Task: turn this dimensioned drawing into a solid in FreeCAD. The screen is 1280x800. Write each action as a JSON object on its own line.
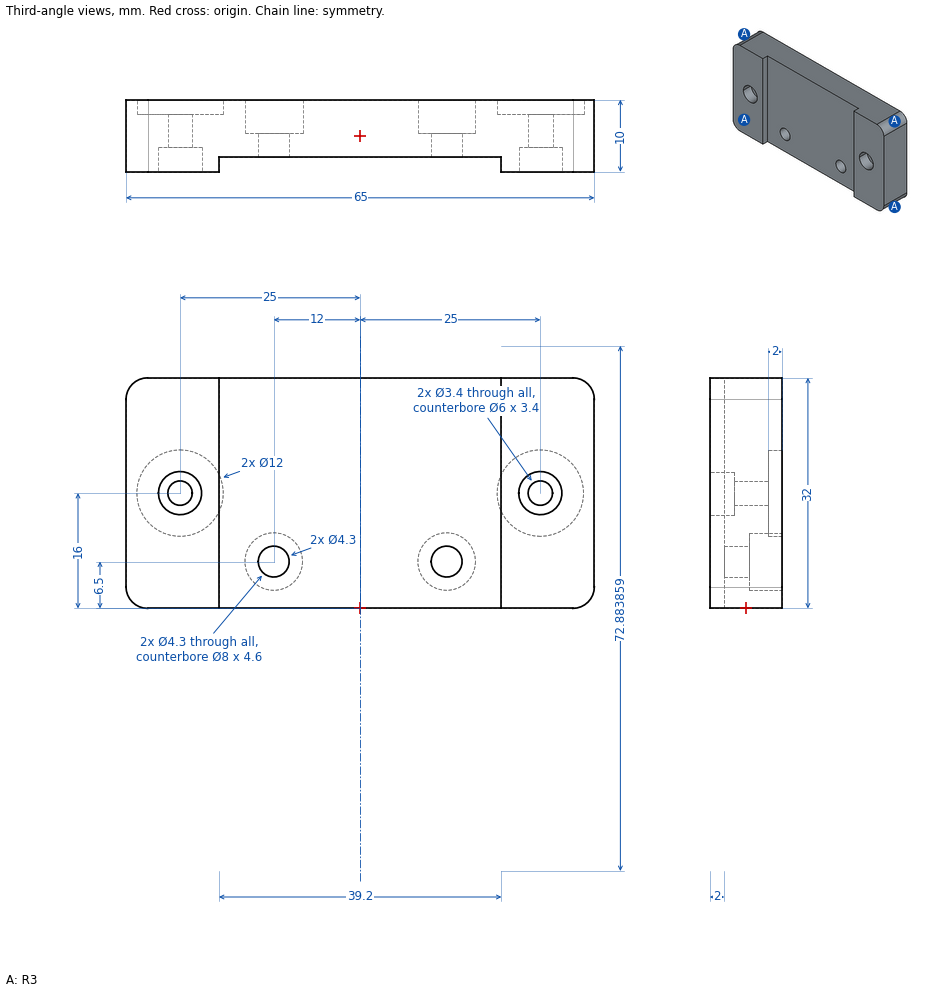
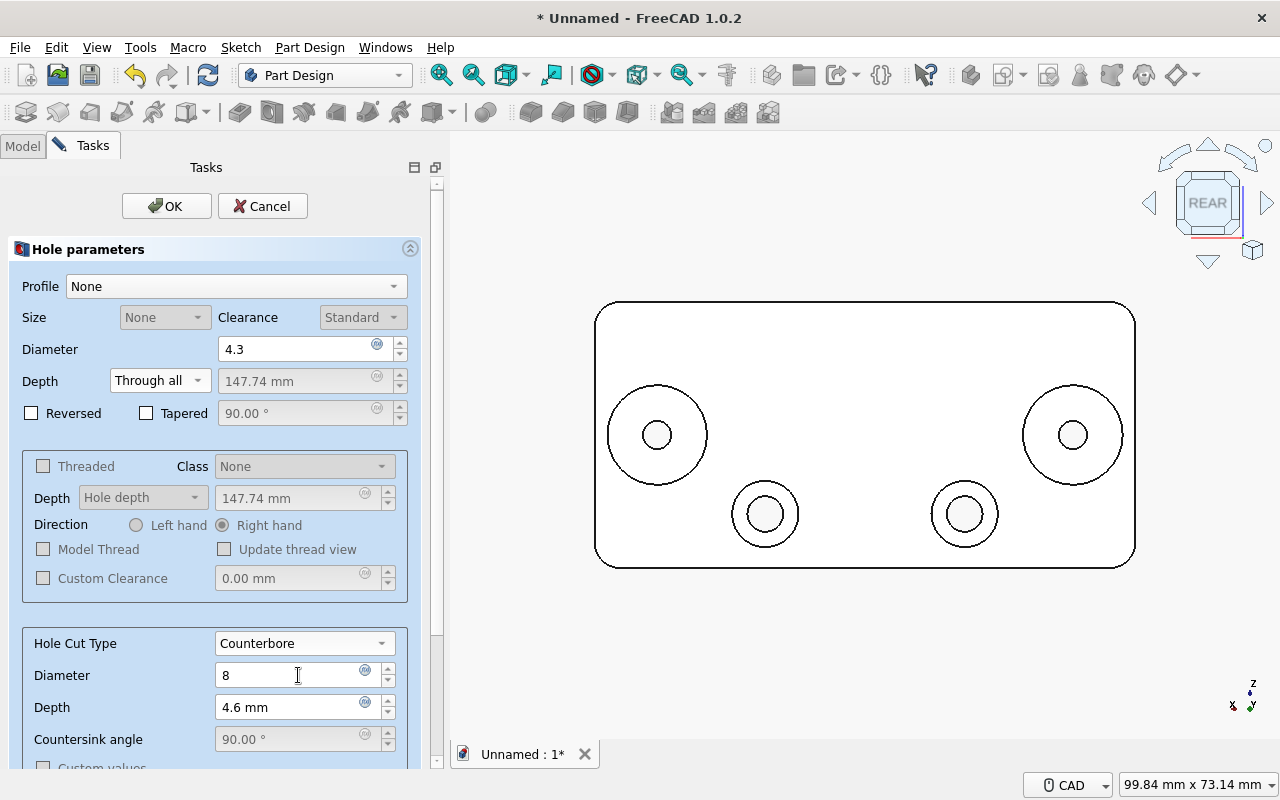
{"action": "left_click", "coordinate": [167, 206]}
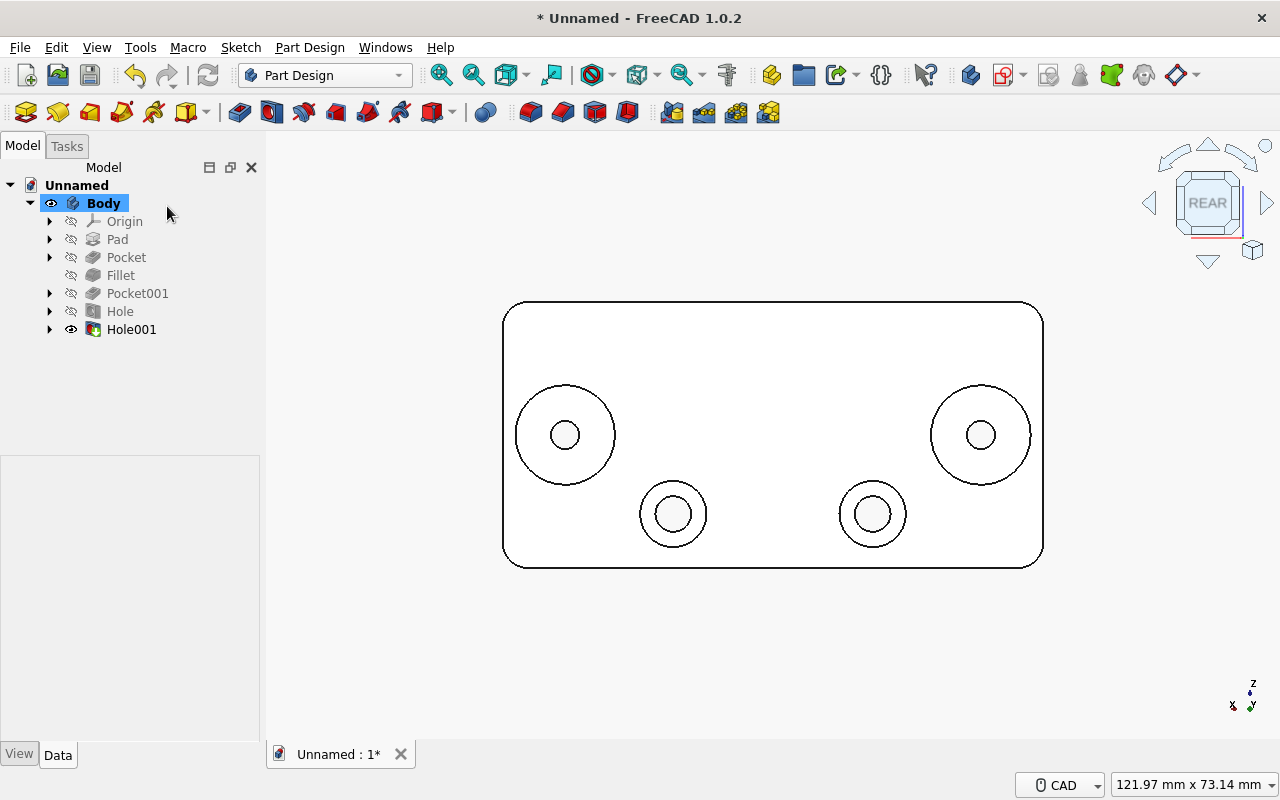
{"action": "key", "text": "0"}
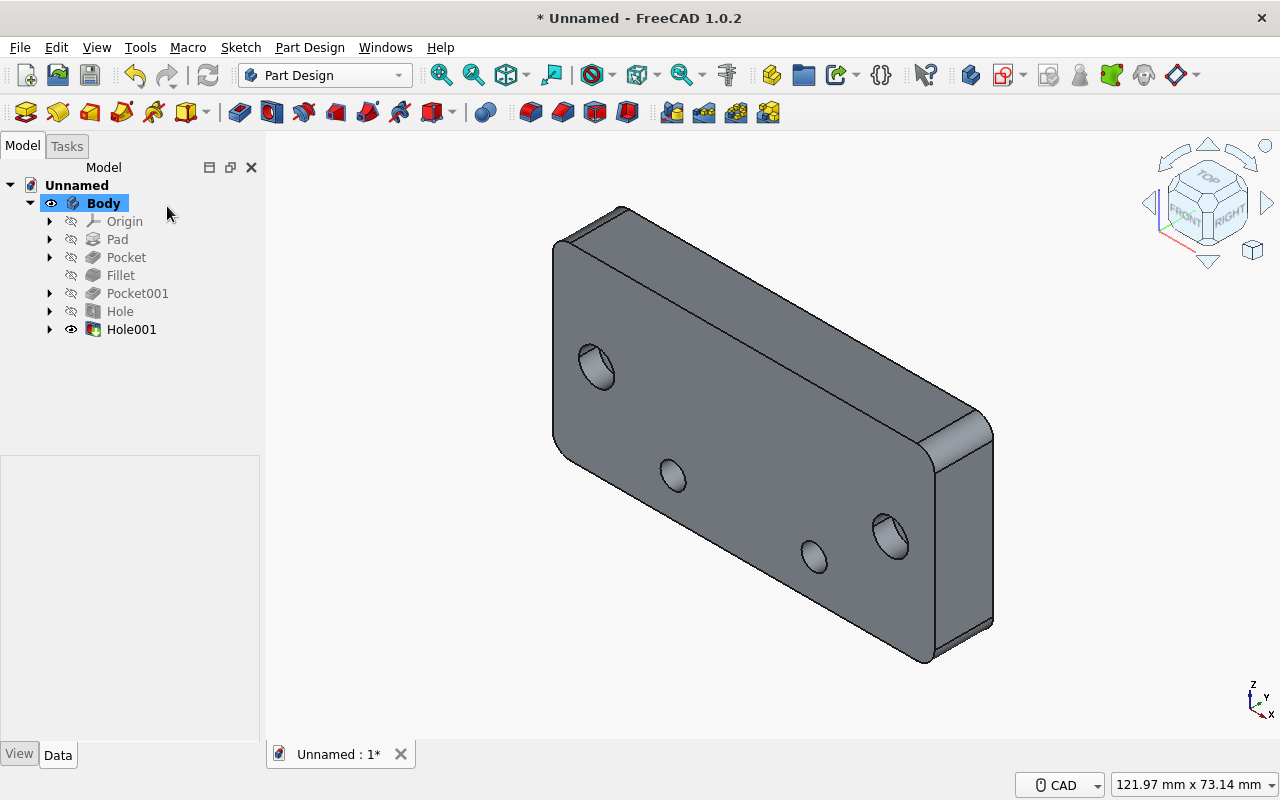
{"action": "left_click", "coordinate": [744, 451]}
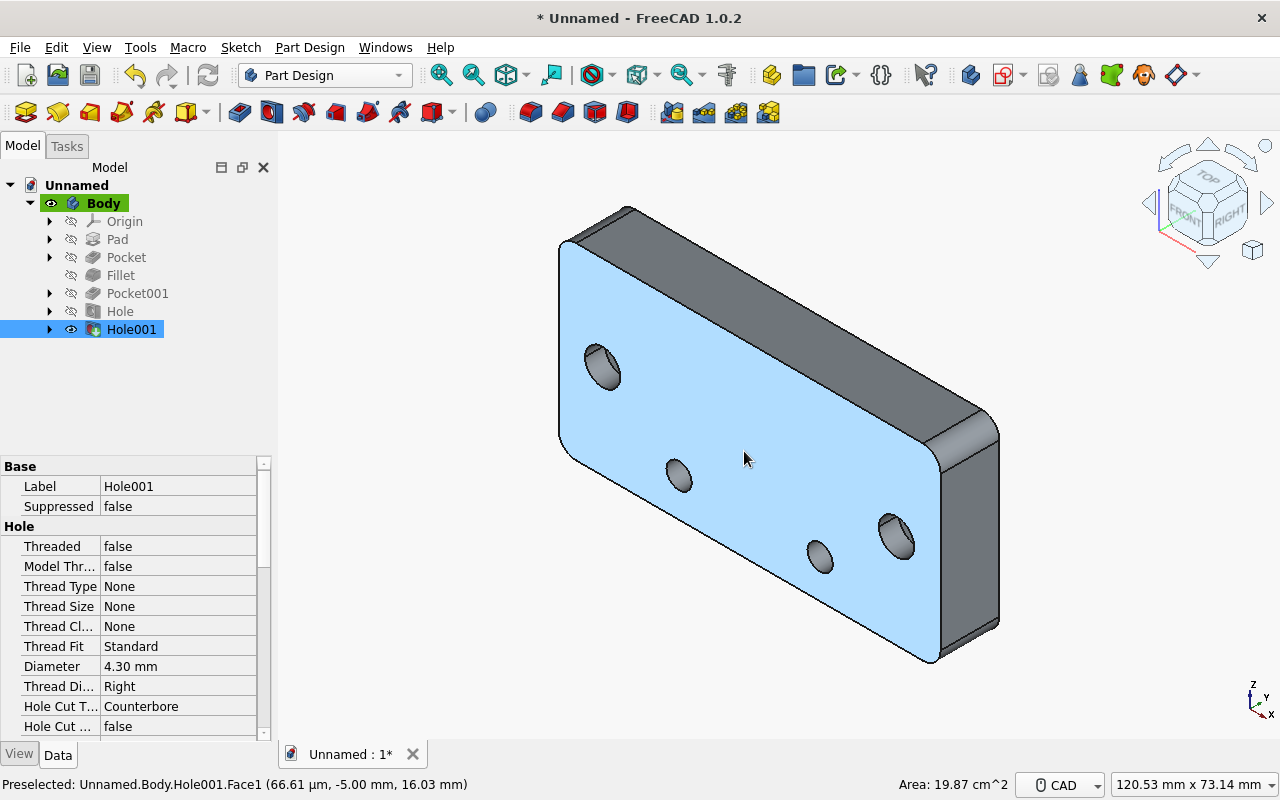
{"action": "left_click", "coordinate": [1004, 76]}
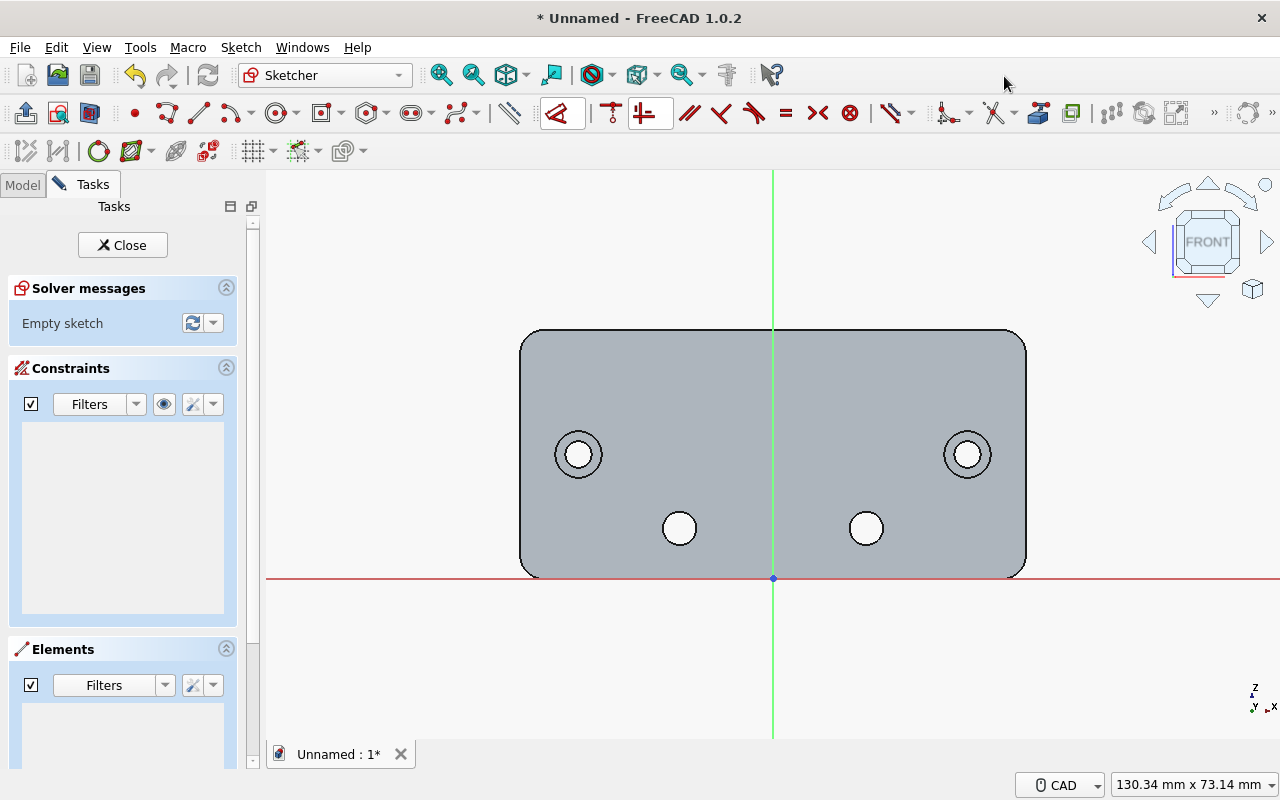
{"action": "scroll", "coordinate": [565, 201], "scroll_direction": "down", "scroll_amount": 2}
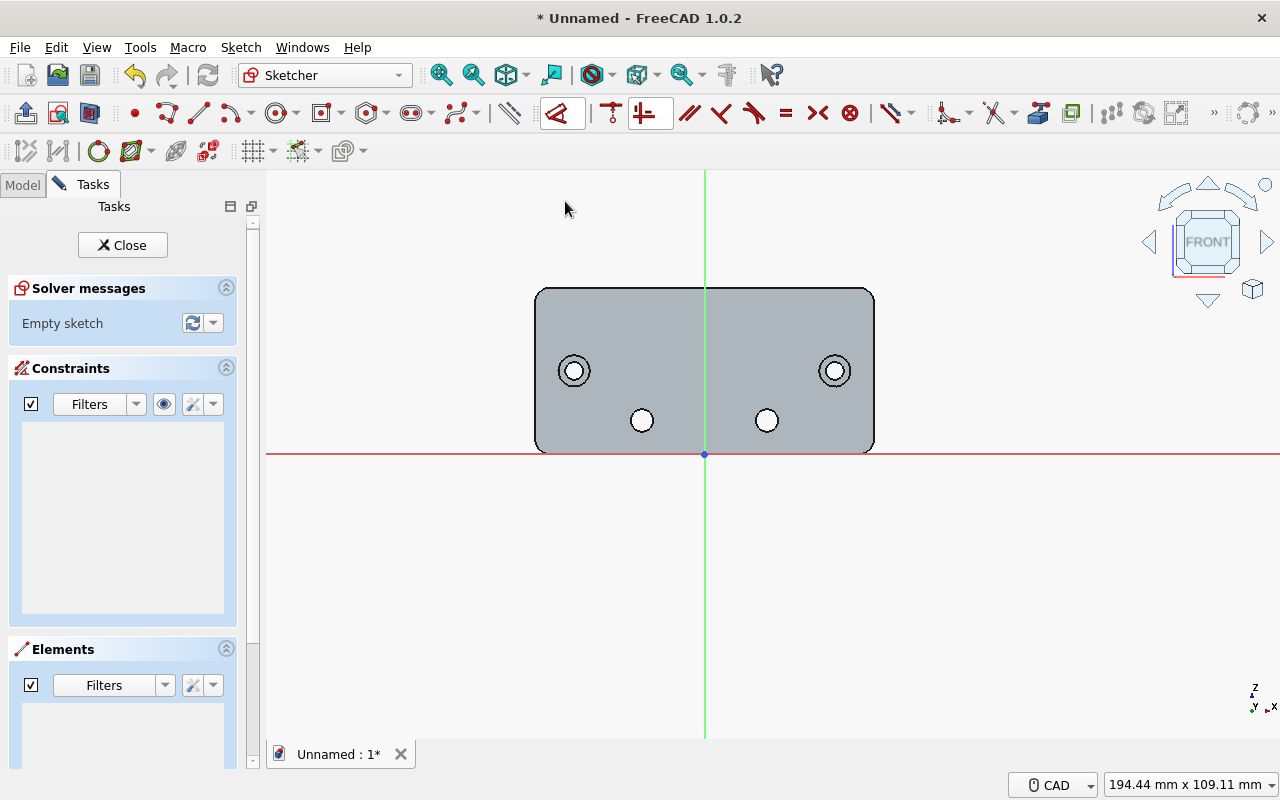
{"action": "left_click", "coordinate": [322, 114]}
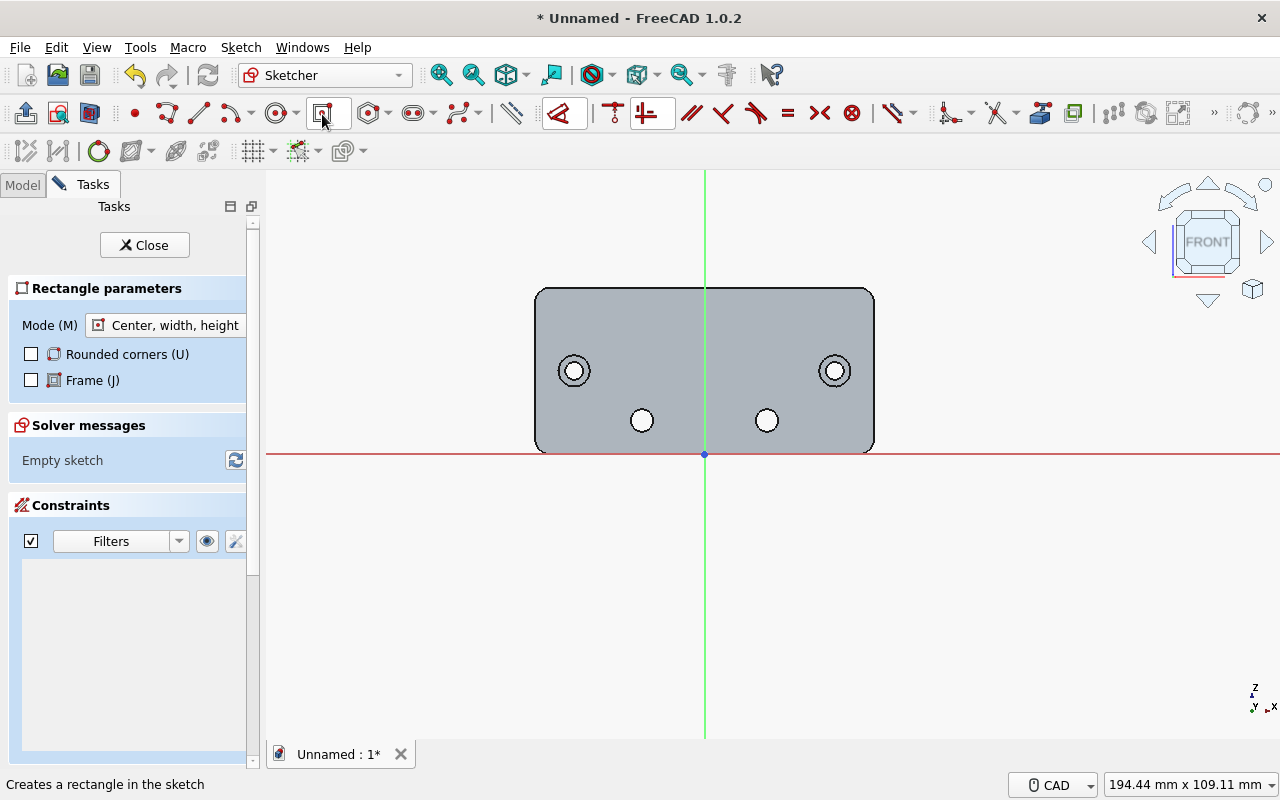
{"action": "left_click", "coordinate": [705, 454]}
{"action": "left_click", "coordinate": [807, 264]}
{"action": "key", "text": "Escape"}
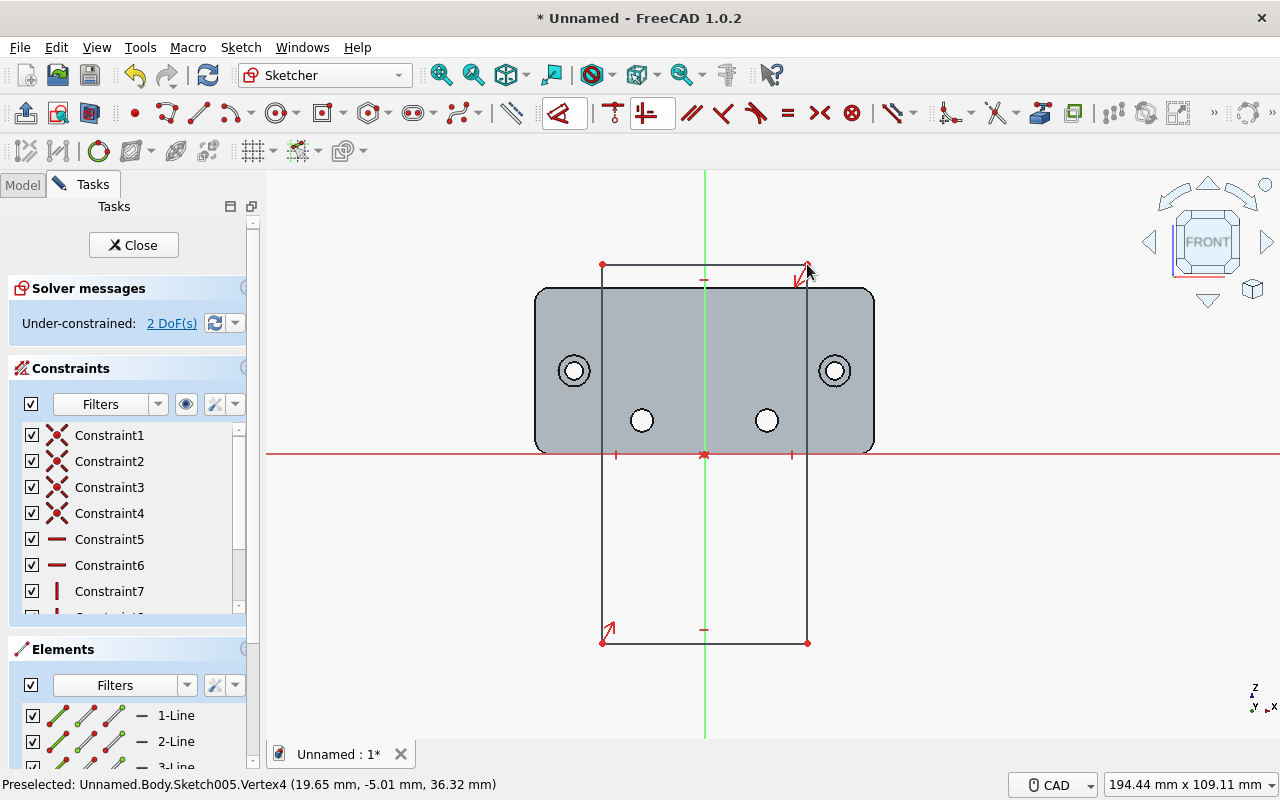
{"action": "left_click", "coordinate": [664, 644]}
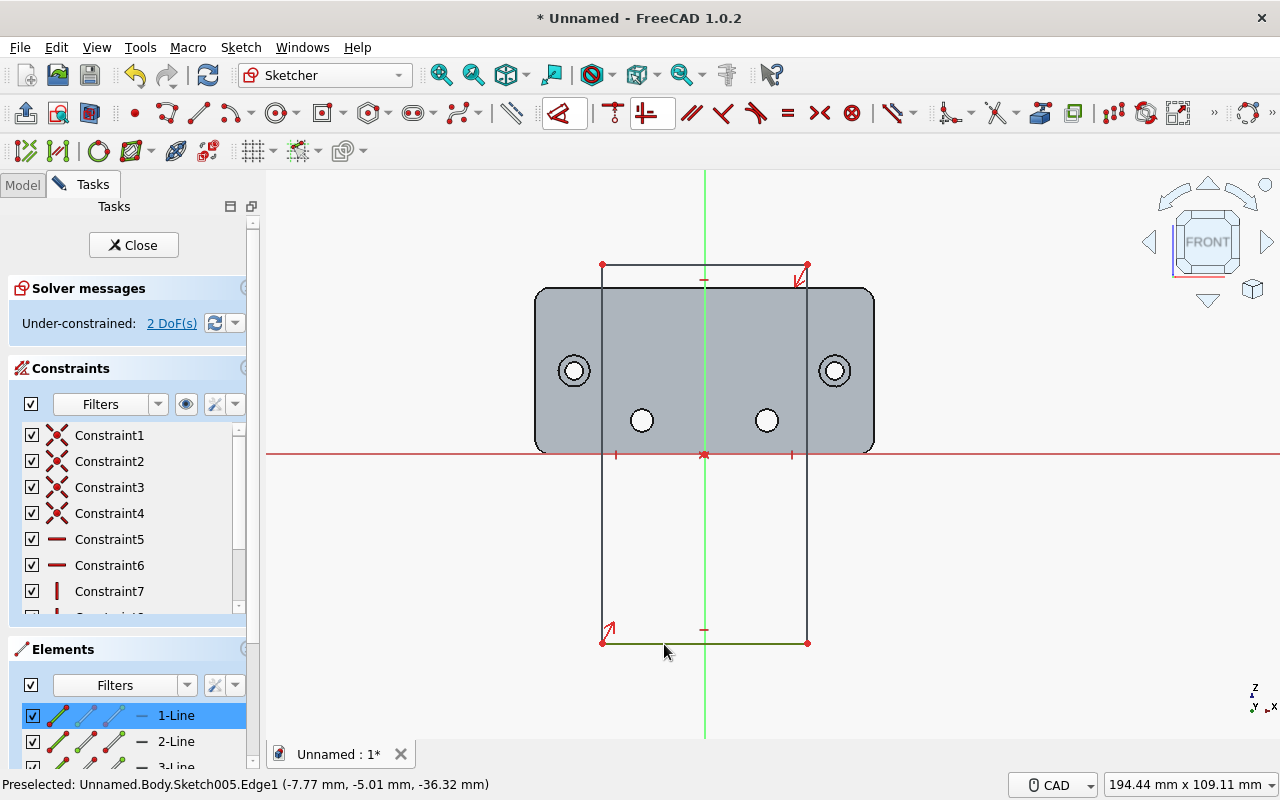
{"action": "key", "text": "l"}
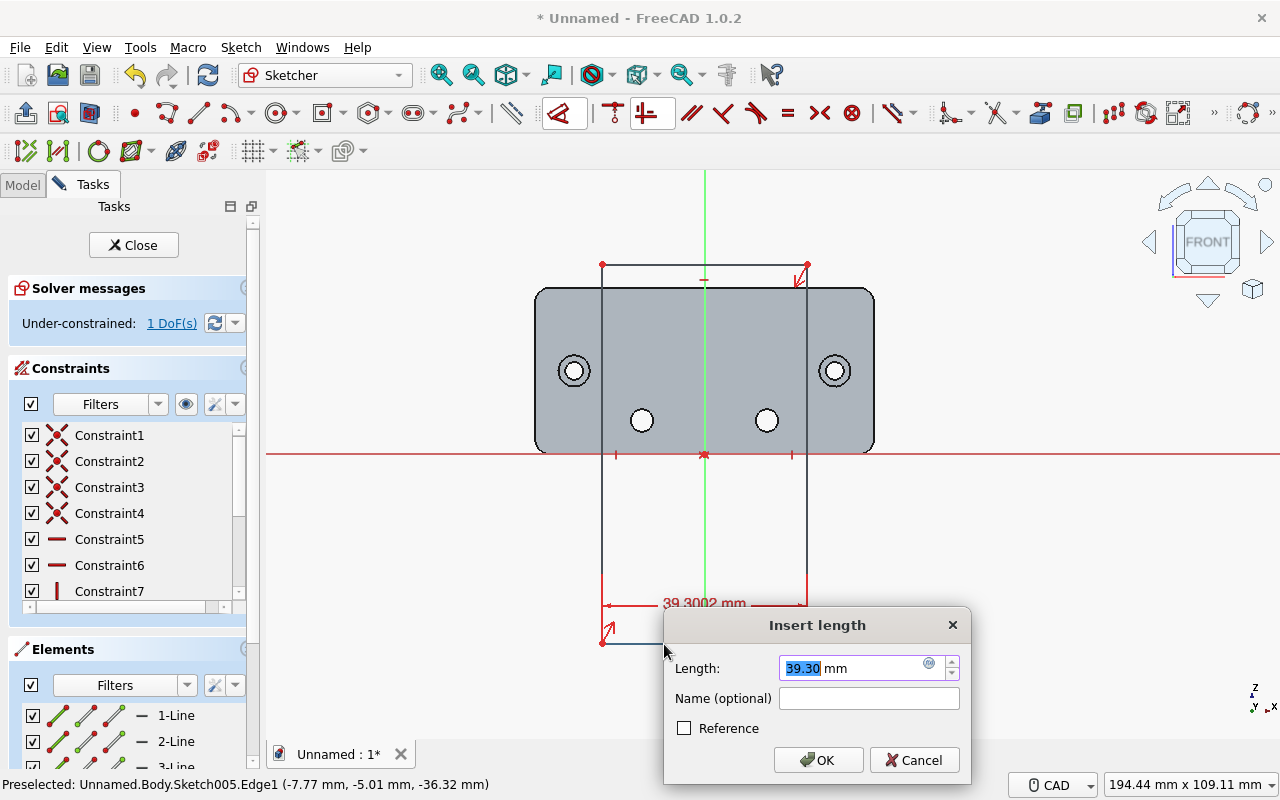
{"action": "type", "text": "39.2"}
{"action": "key", "text": "Return"}